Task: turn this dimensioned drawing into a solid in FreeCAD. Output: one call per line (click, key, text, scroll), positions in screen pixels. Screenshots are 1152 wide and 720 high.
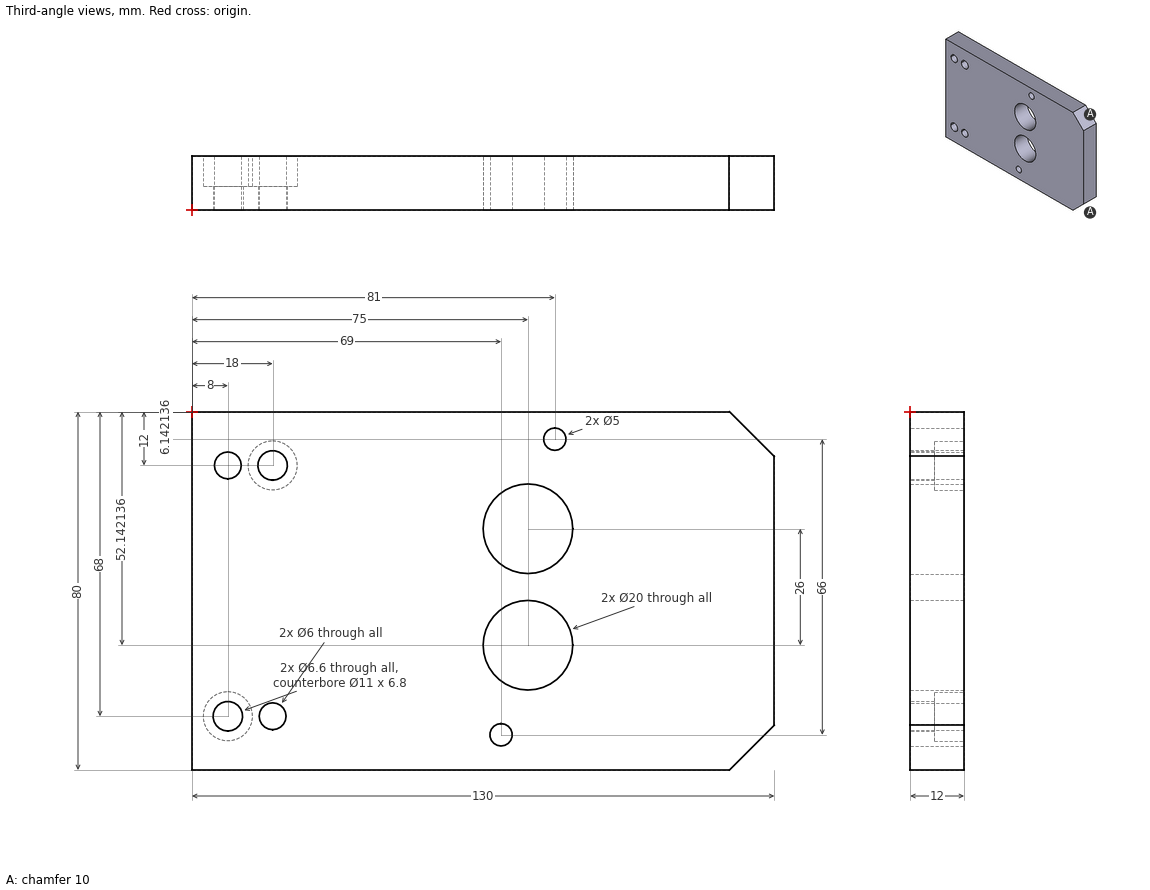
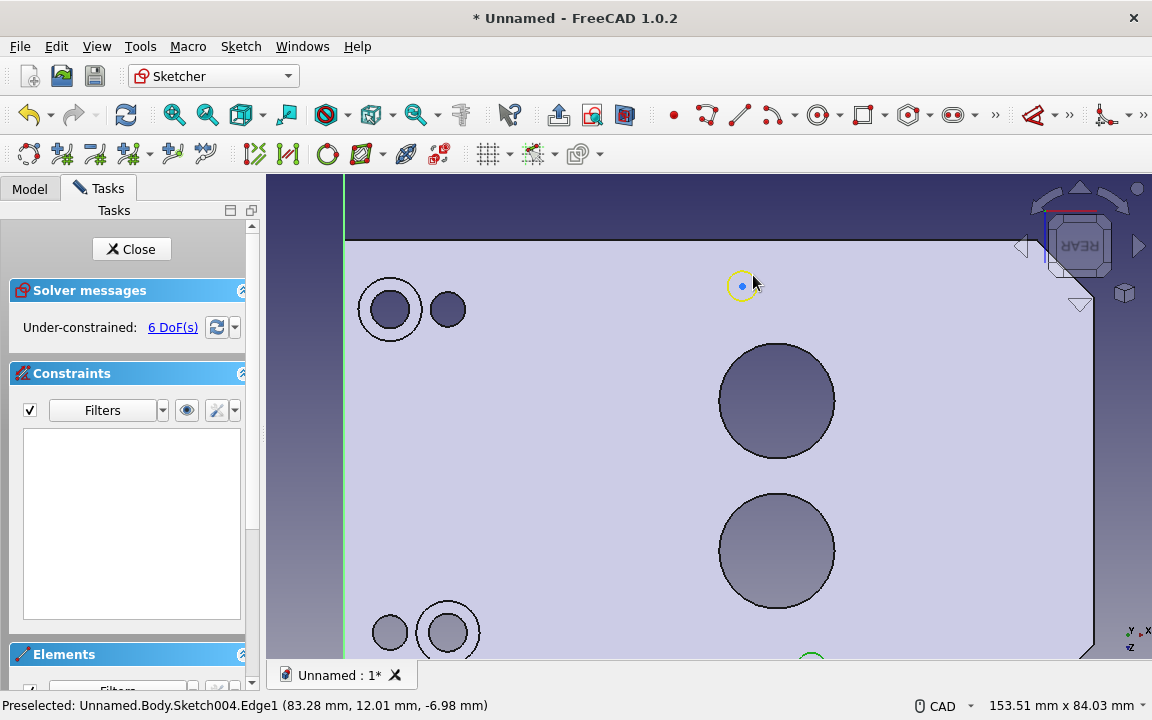
click(753, 276)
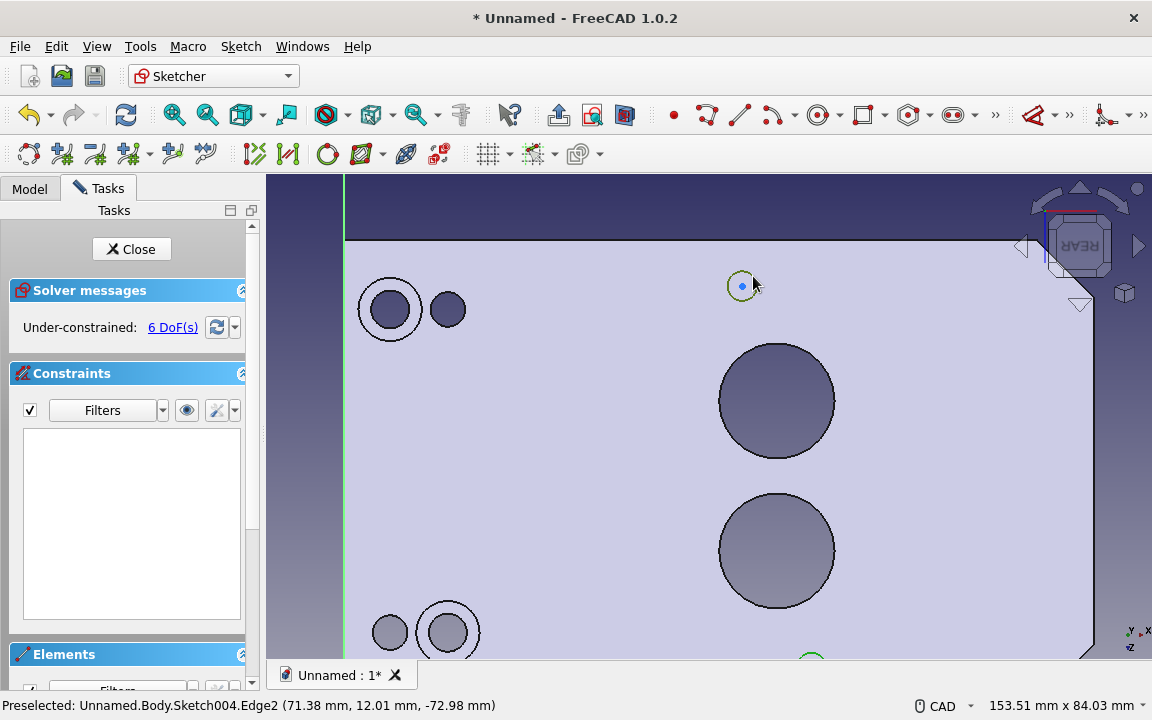
key(e)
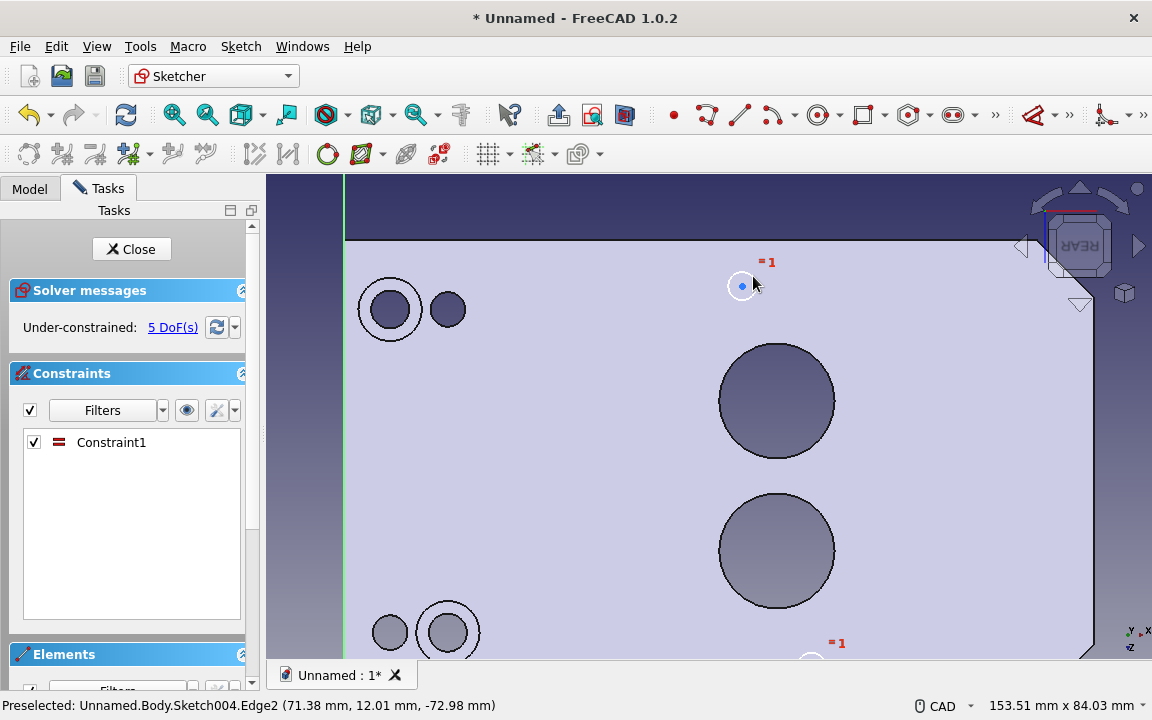
key(d)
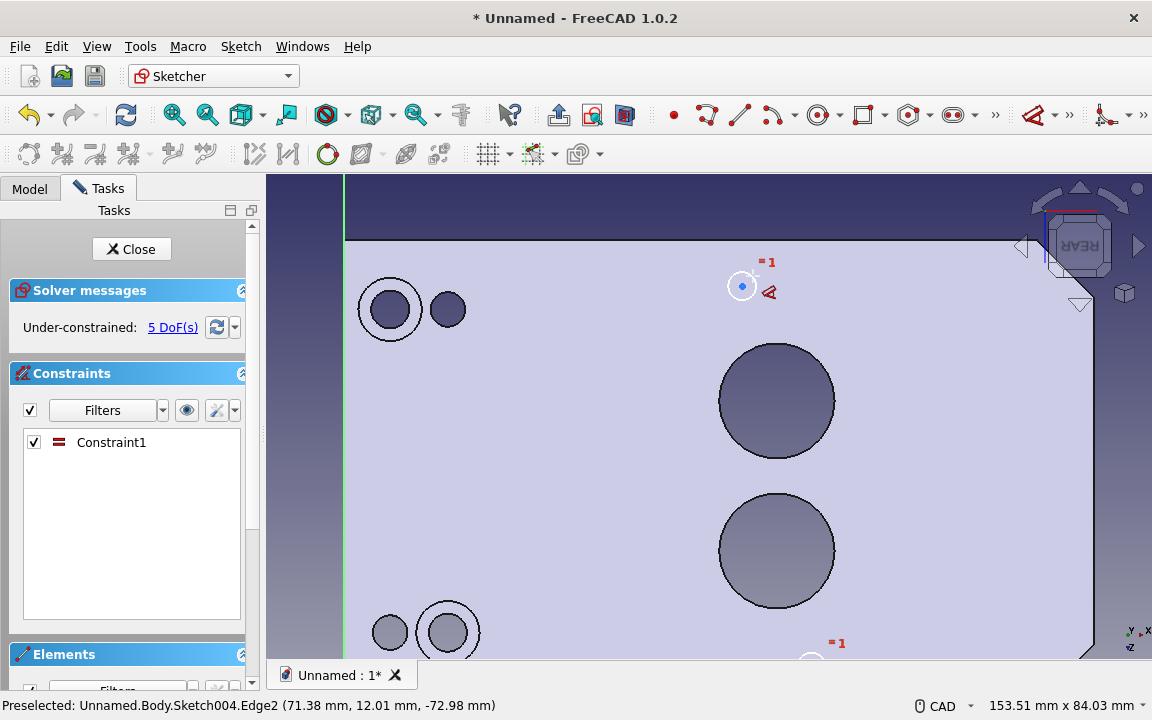
scroll(753, 274, down, 2)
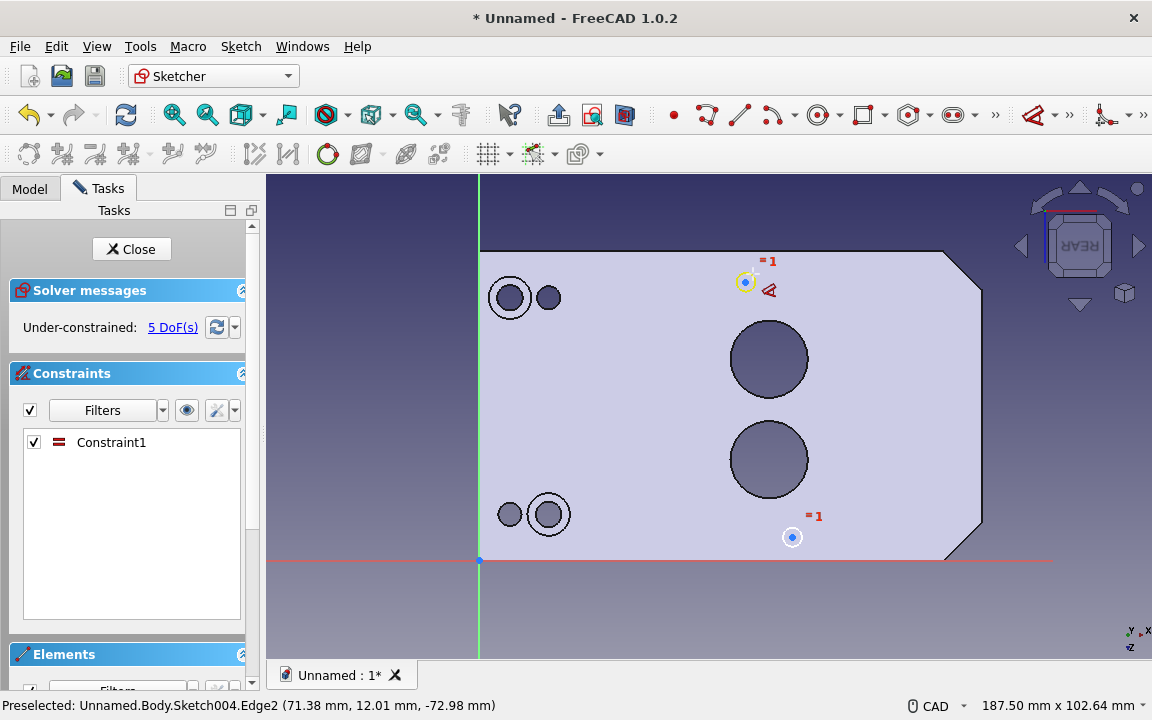
scroll(799, 531, up, 4)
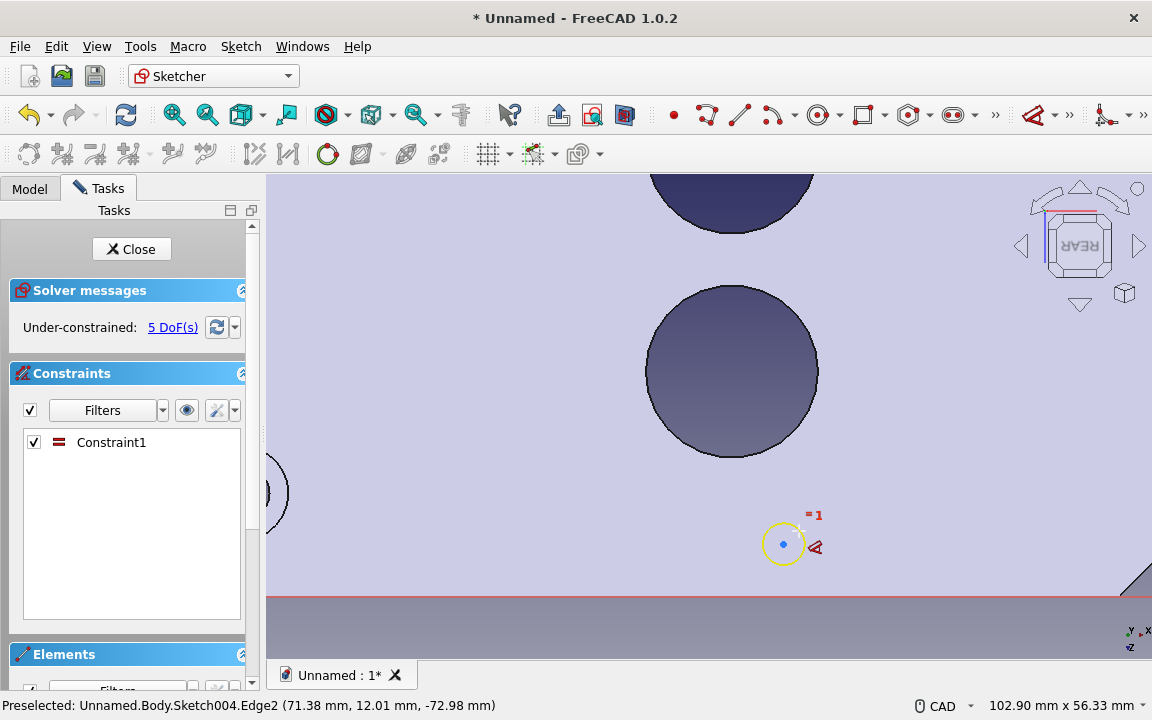
click(799, 529)
click(822, 506)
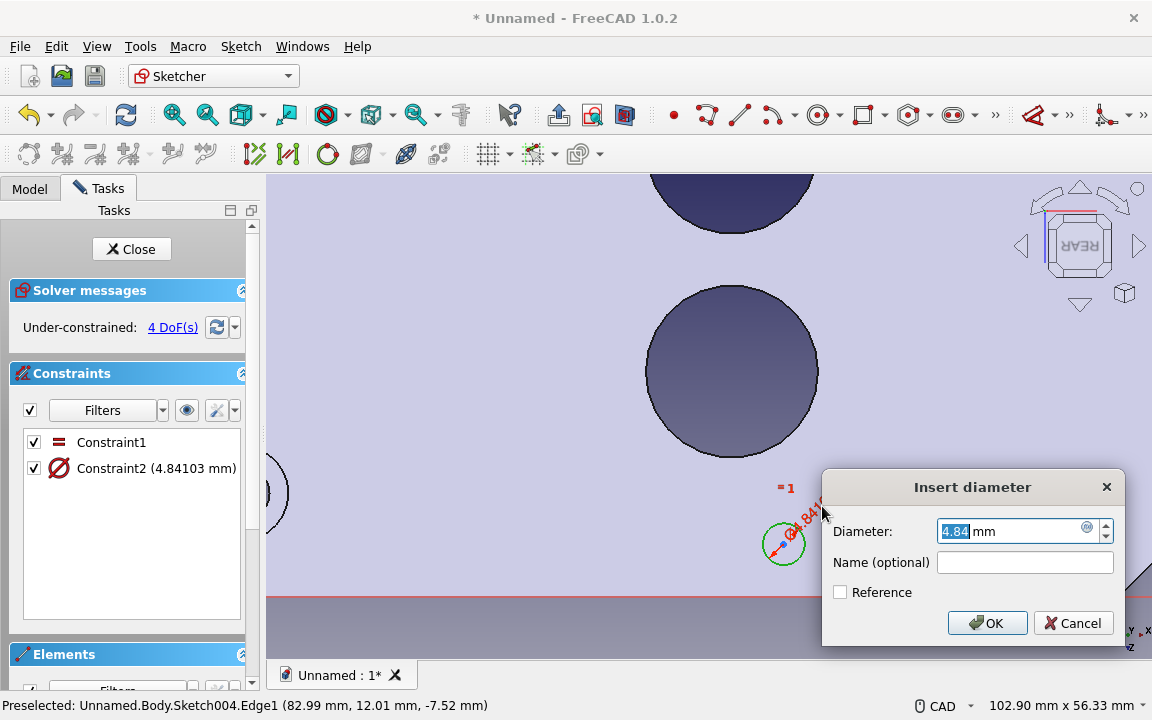
text(5)
key(Return)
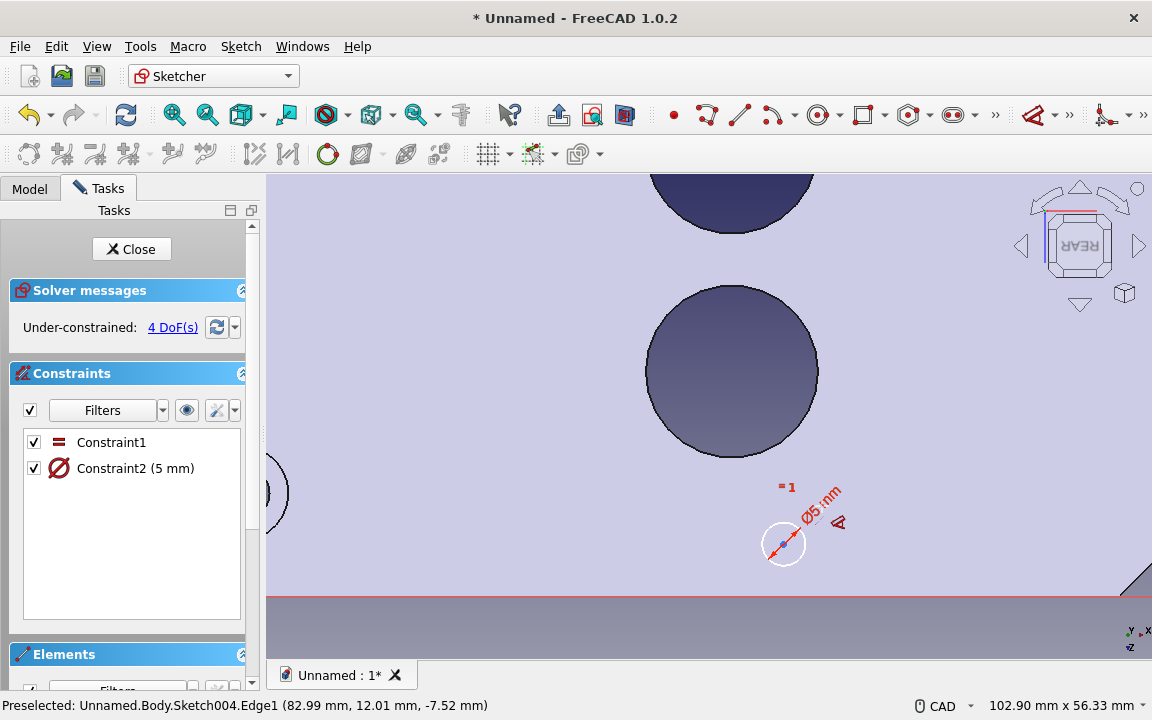
click(784, 544)
click(539, 631)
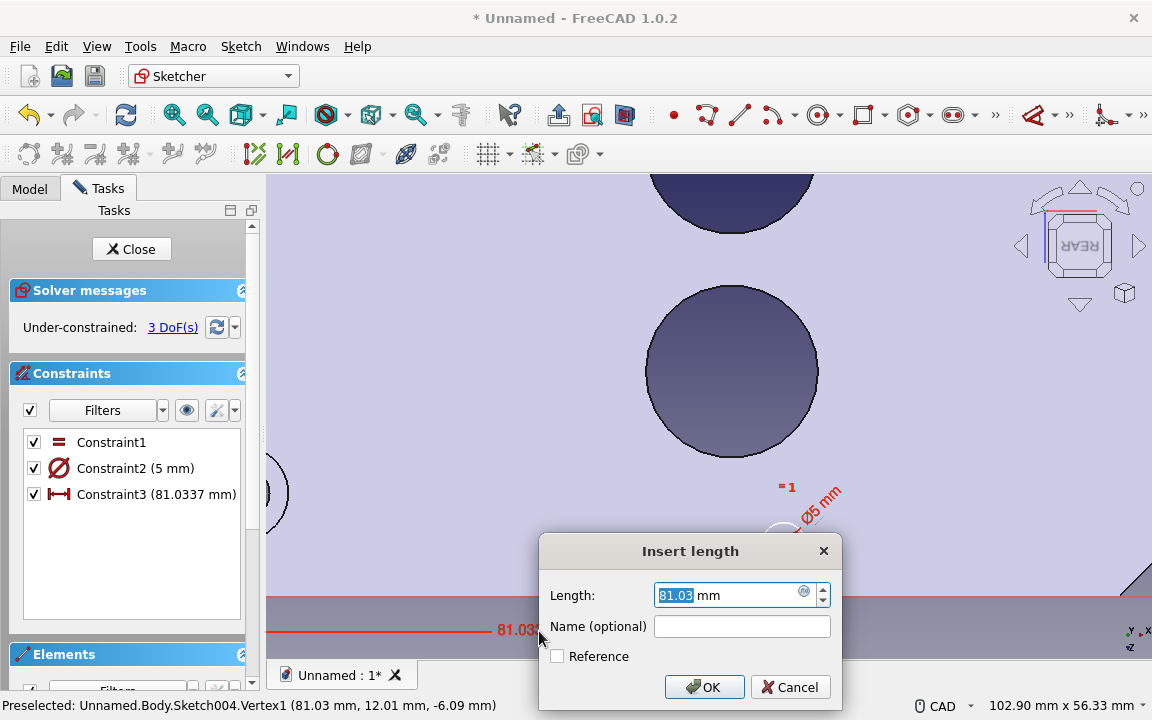
text(81)
key(Return)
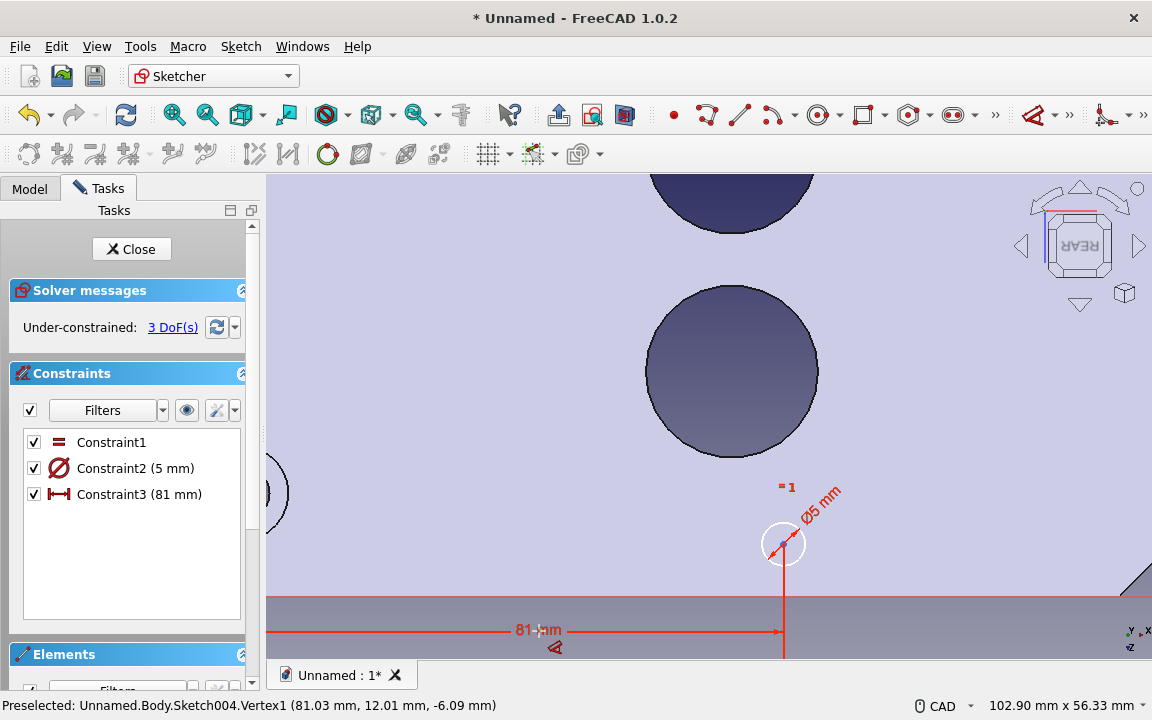
scroll(800, 532, down, 4)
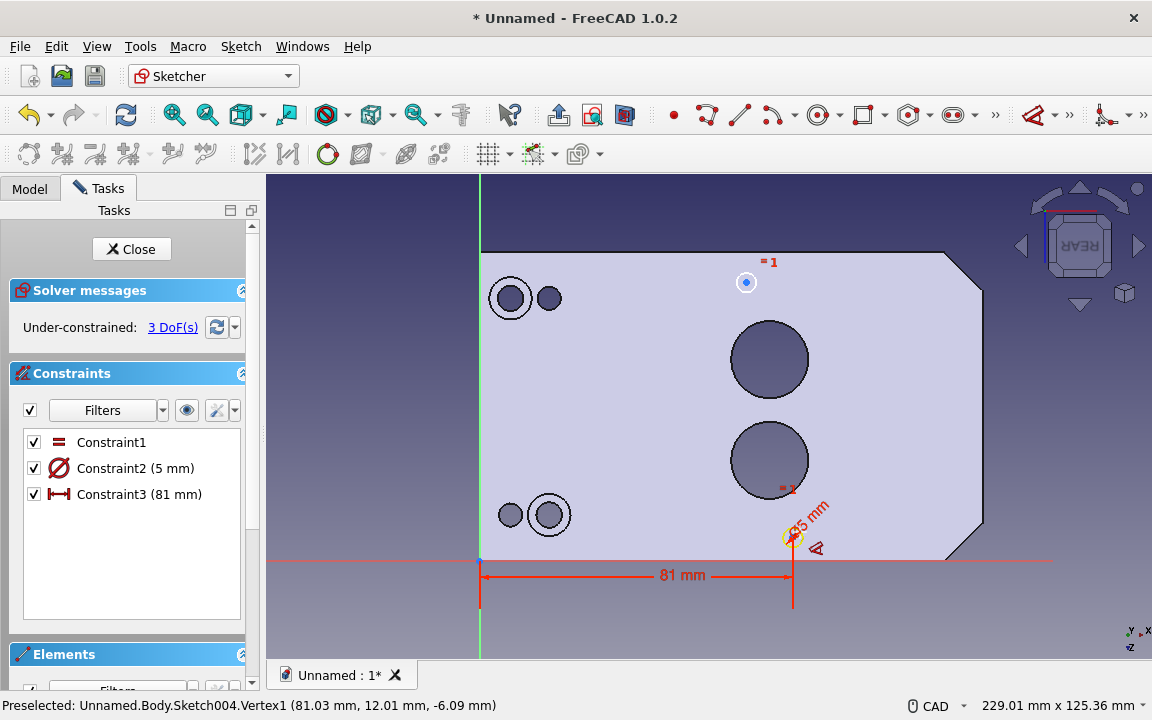
click(747, 283)
click(552, 595)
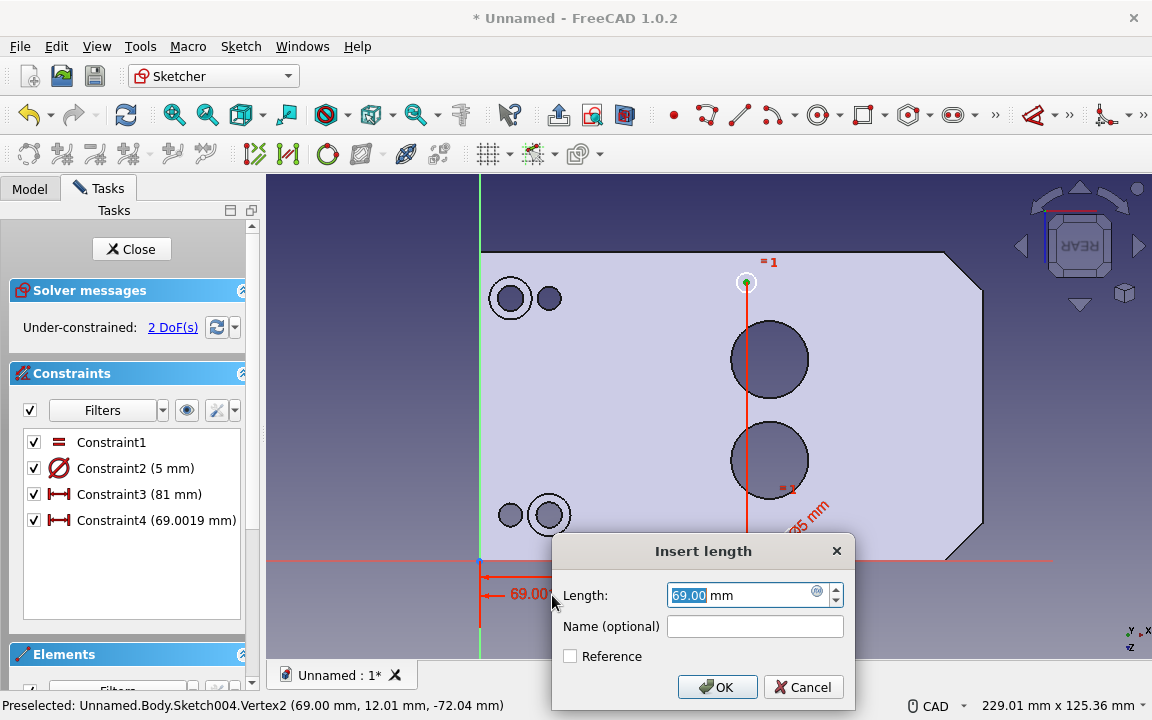
text(69)
key(Return)